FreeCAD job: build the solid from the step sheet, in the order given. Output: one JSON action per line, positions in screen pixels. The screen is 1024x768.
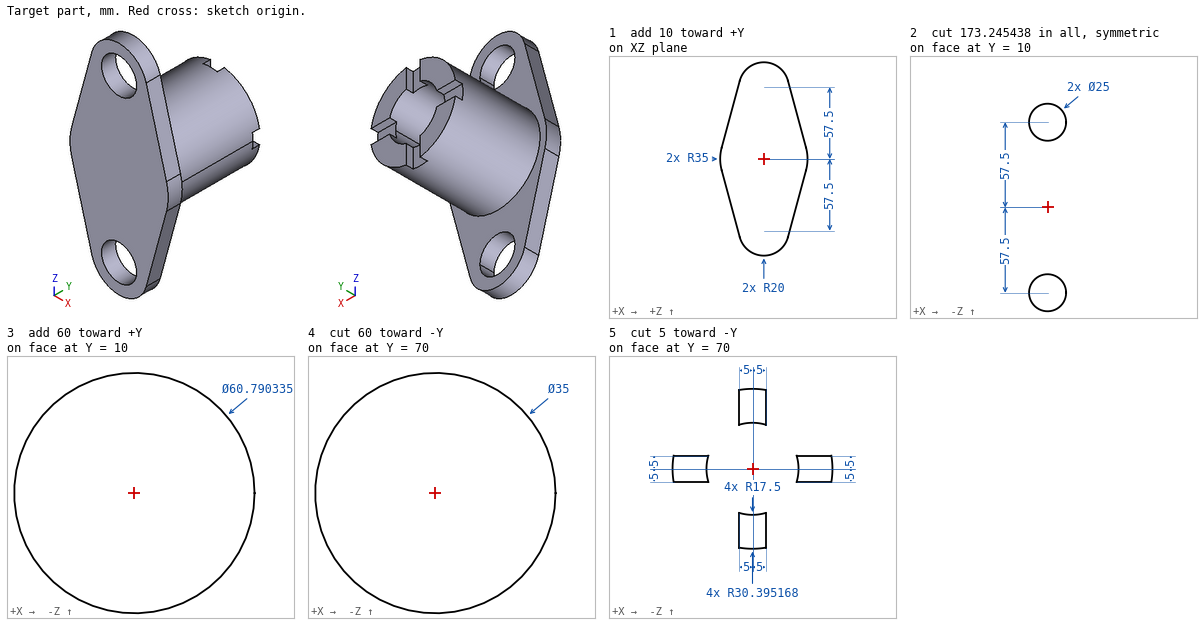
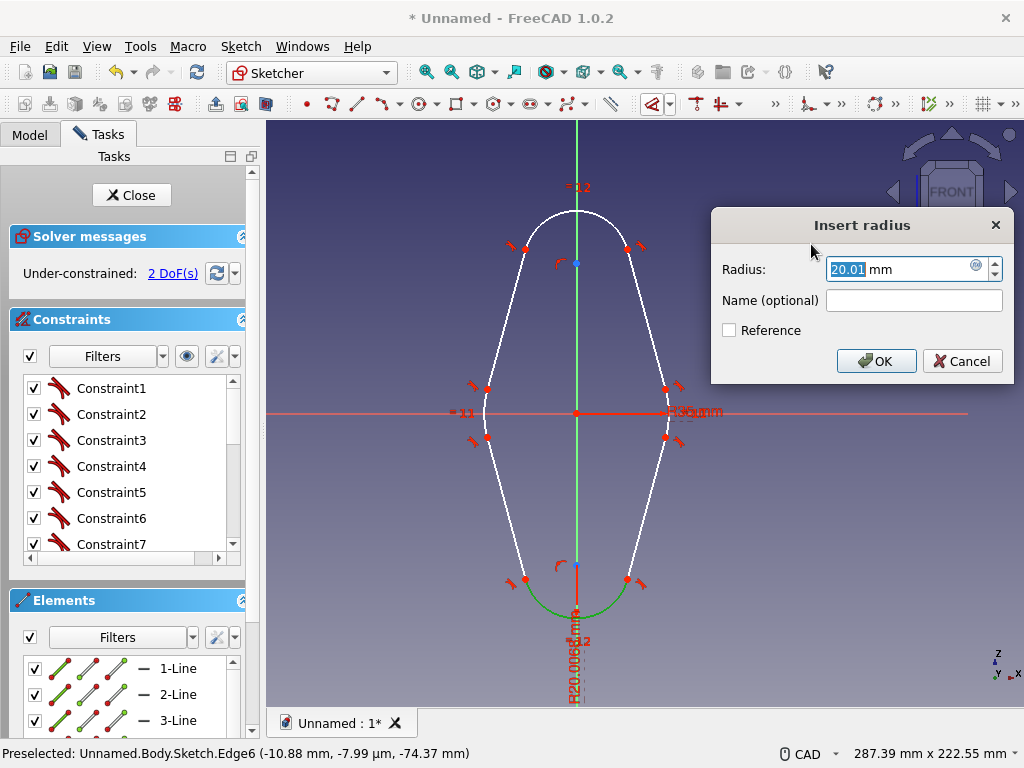
{"action": "type", "text": "20"}
{"action": "key", "text": "Return"}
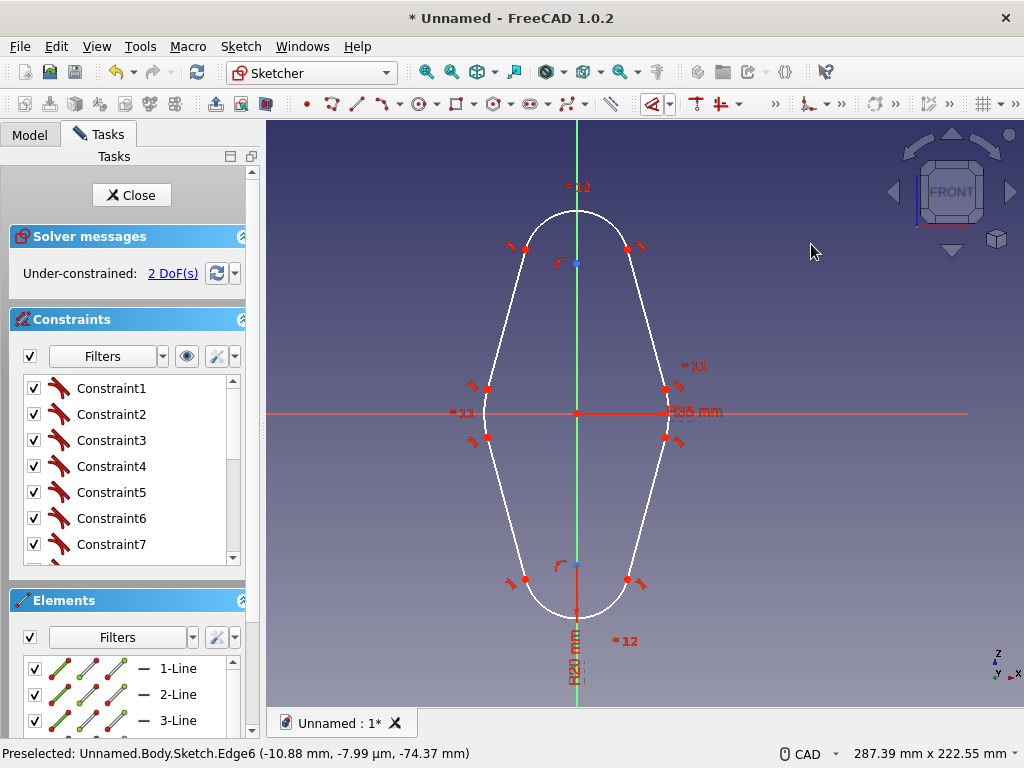
{"action": "left_click", "coordinate": [577, 566]}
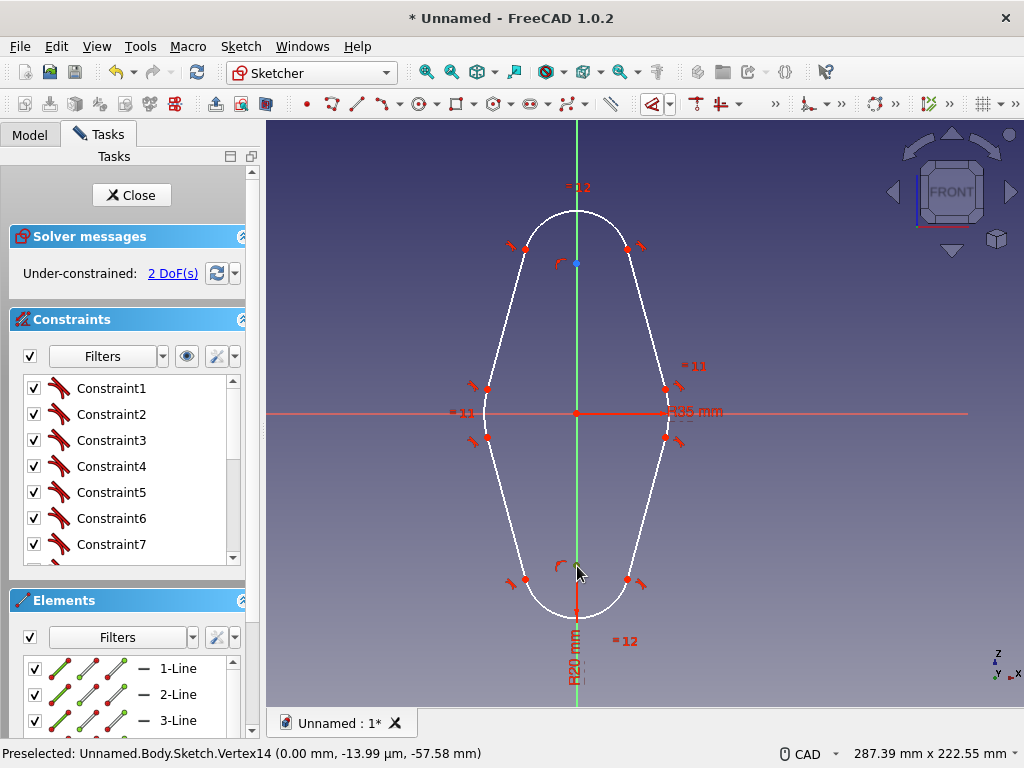
{"action": "left_click", "coordinate": [670, 104]}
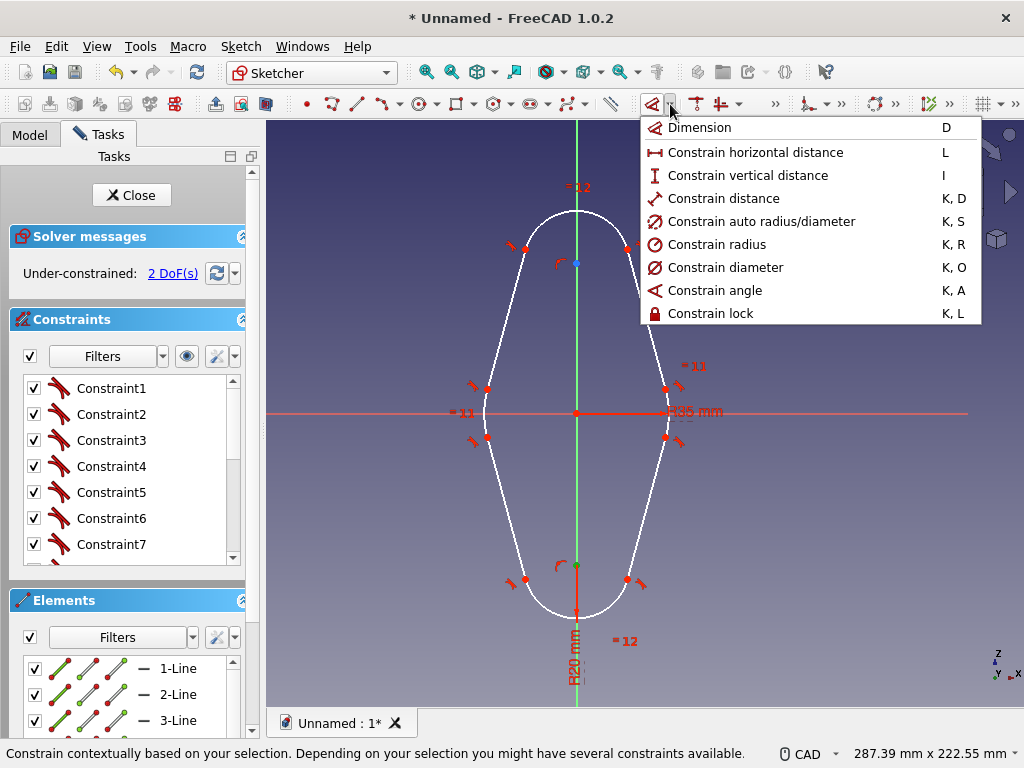
{"action": "left_click", "coordinate": [811, 176]}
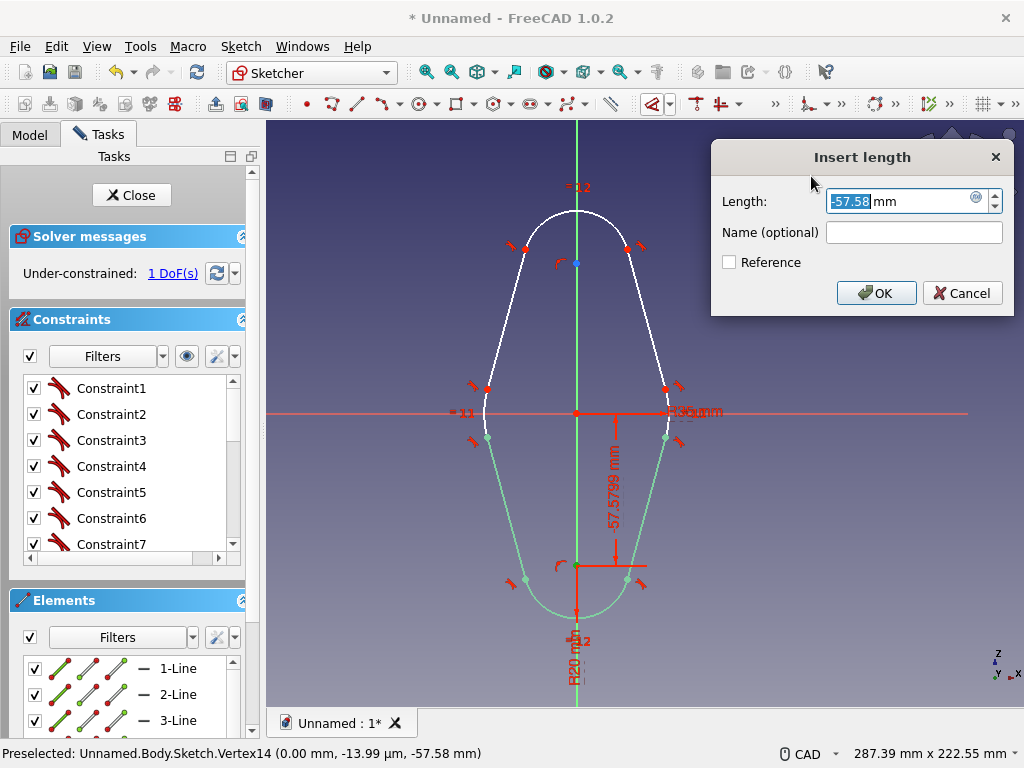
{"action": "type", "text": "-57.5"}
{"action": "key", "text": "Return"}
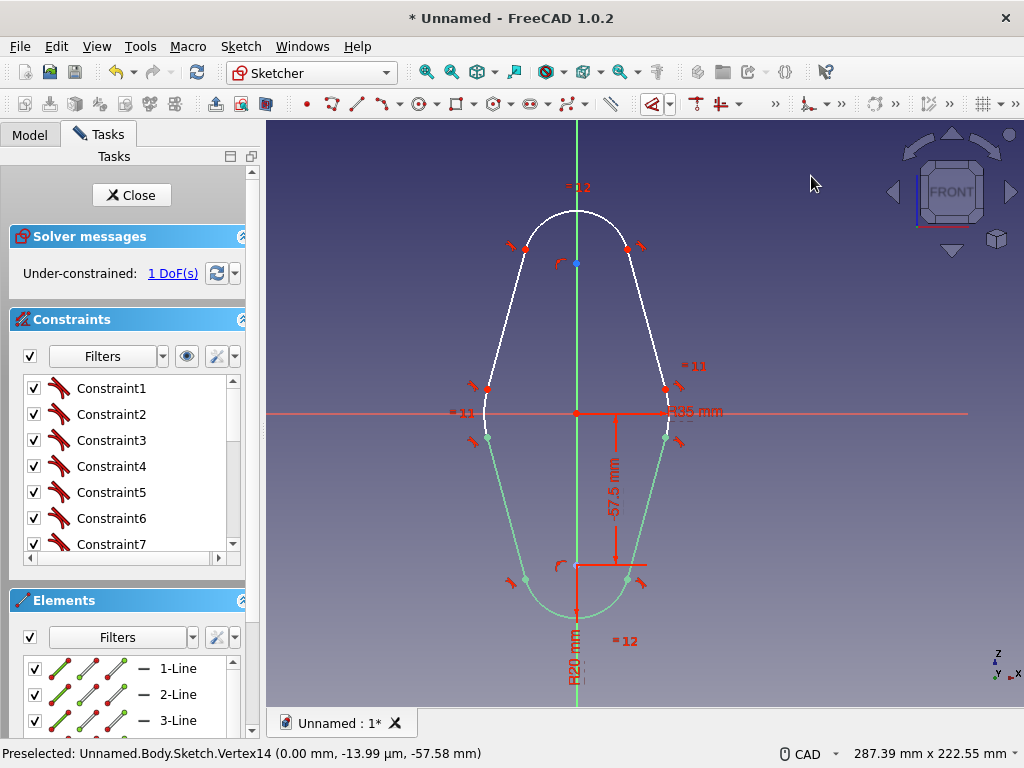
{"action": "left_click", "coordinate": [577, 264]}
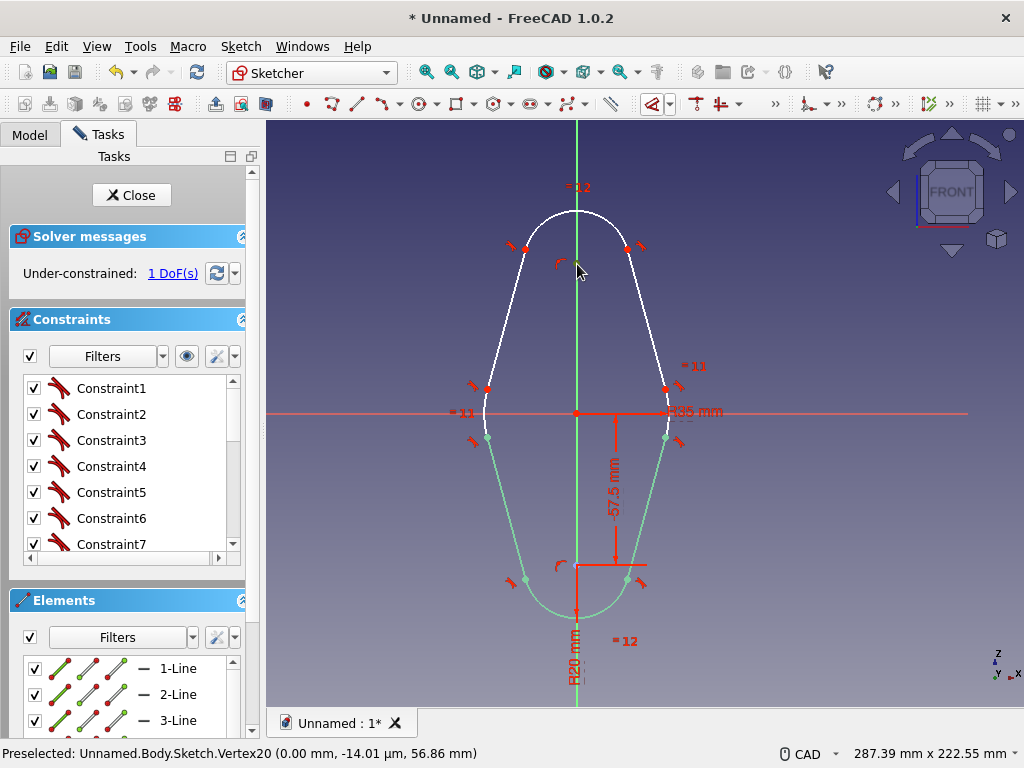
{"action": "key", "text": "i"}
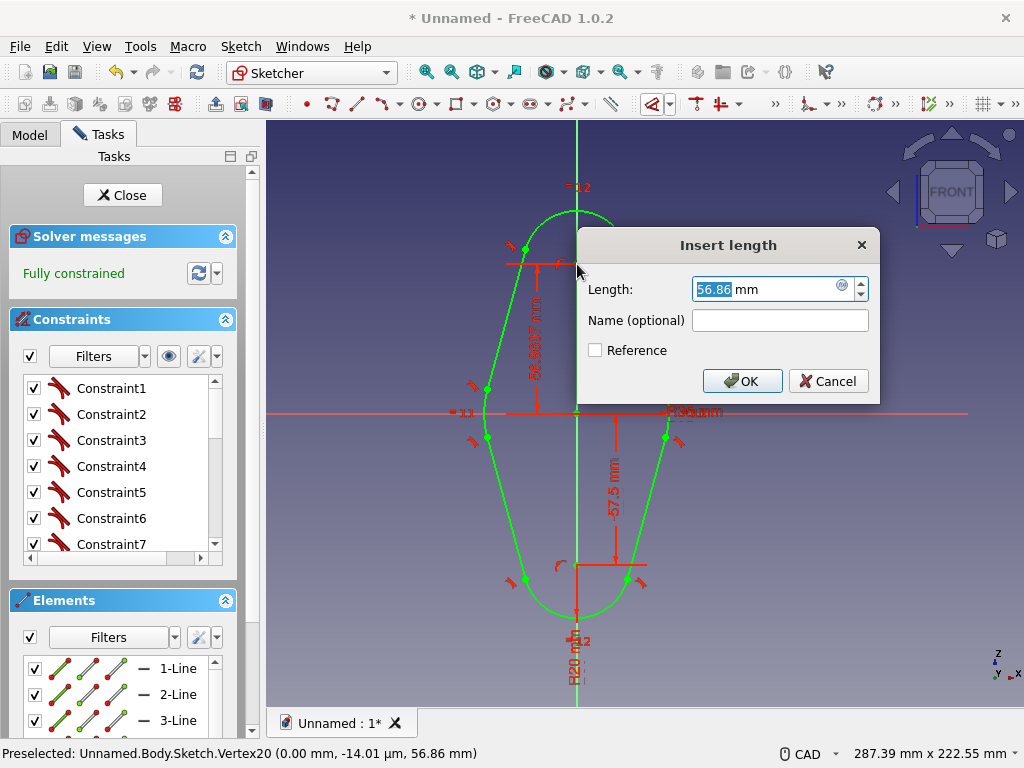
{"action": "type", "text": "57.5"}
{"action": "key", "text": "Return"}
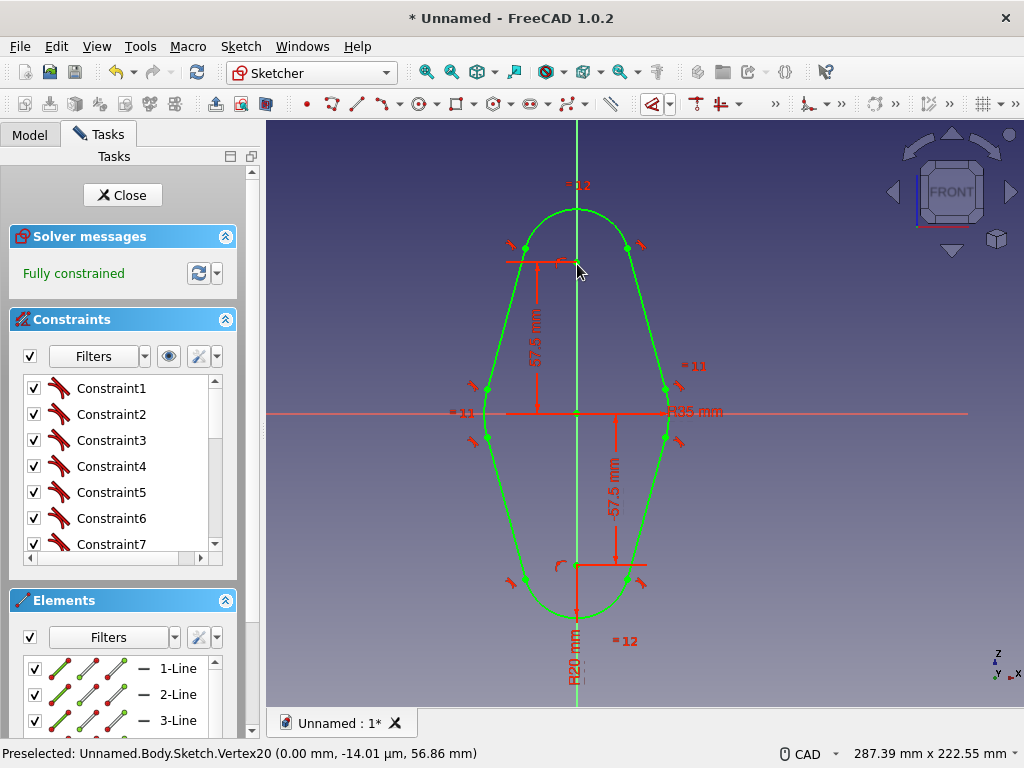
{"action": "left_click", "coordinate": [123, 195]}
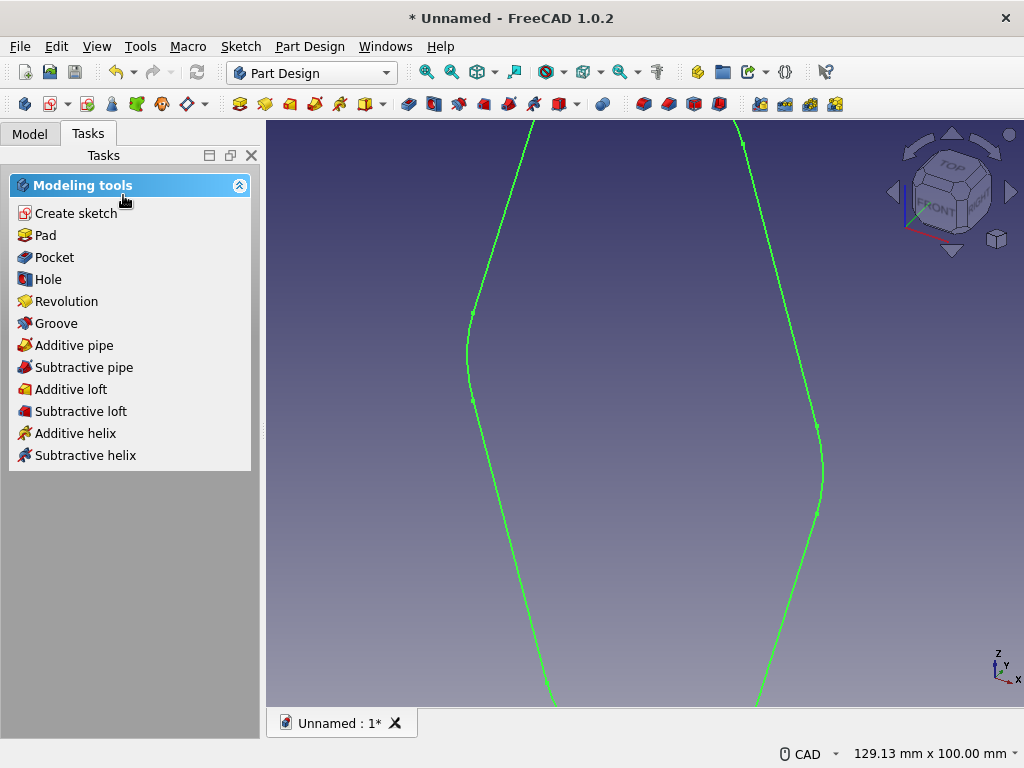
{"action": "left_click", "coordinate": [240, 104]}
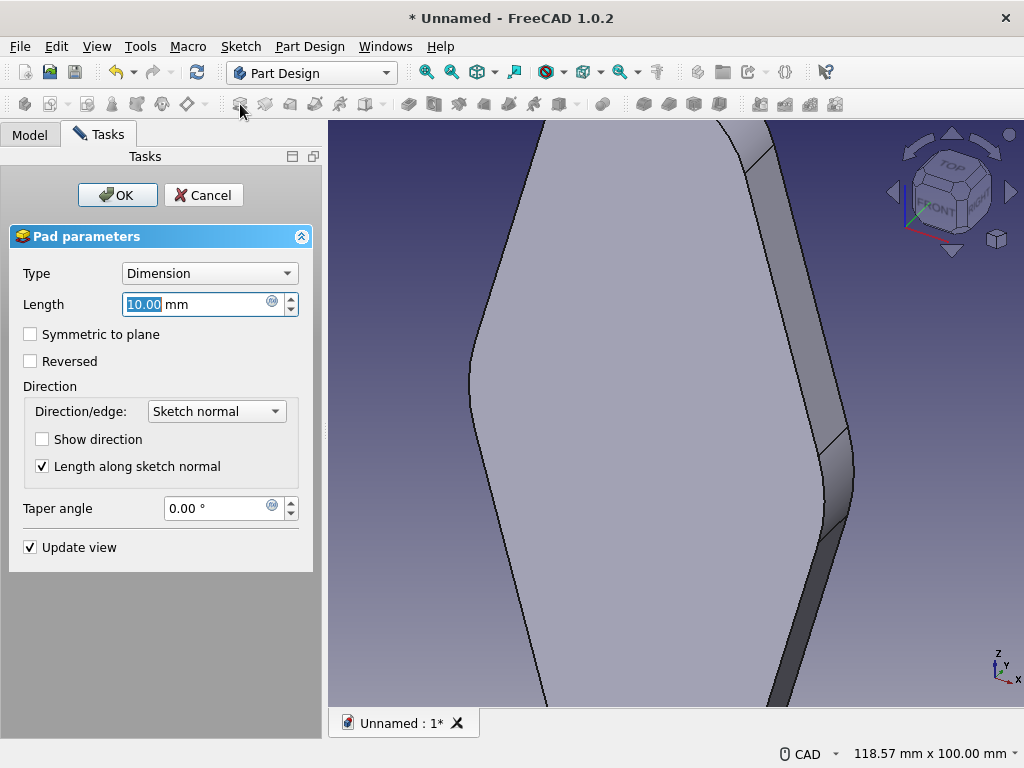
{"action": "type", "text": "10"}
{"action": "key", "text": "Tab"}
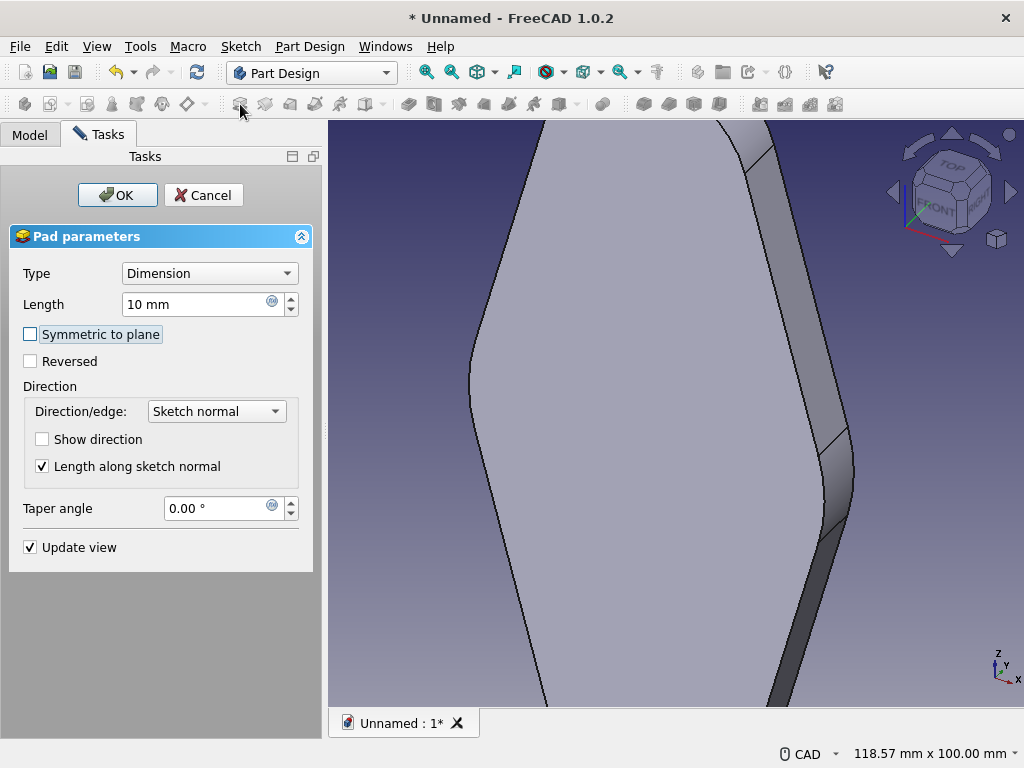
{"action": "left_click", "coordinate": [31, 361]}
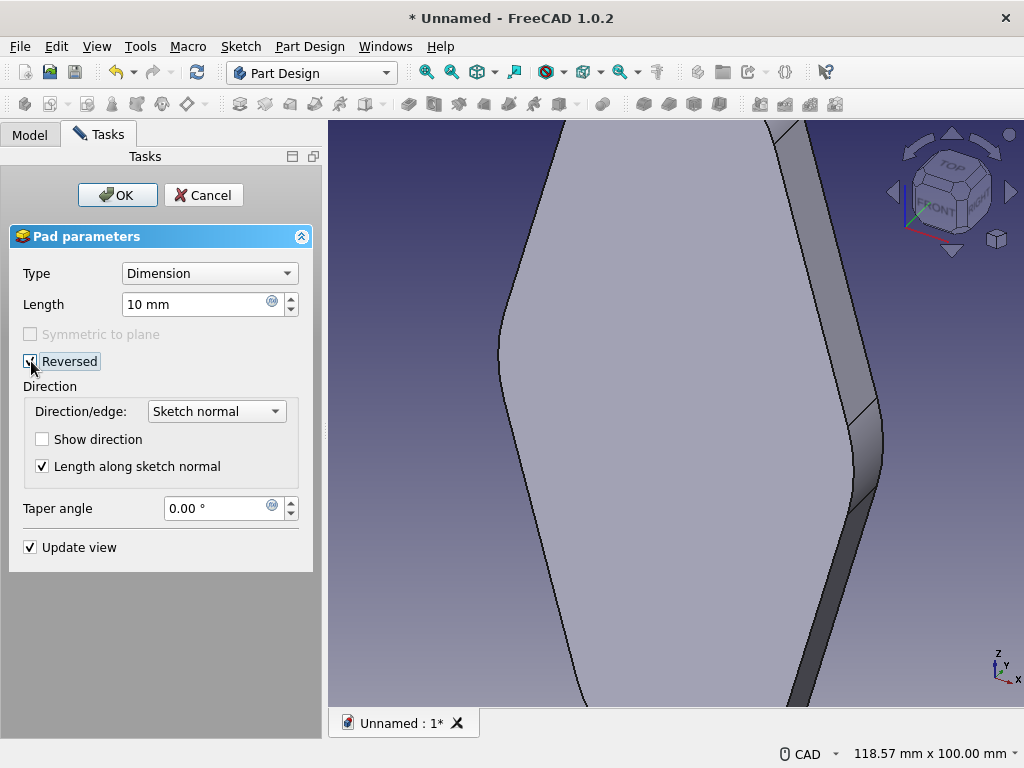
{"action": "left_click", "coordinate": [118, 195]}